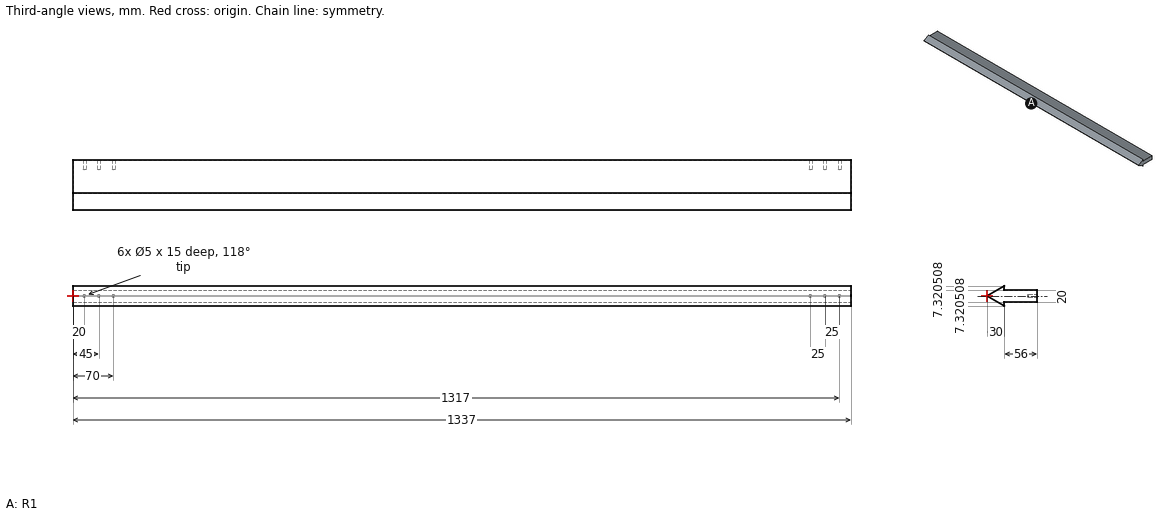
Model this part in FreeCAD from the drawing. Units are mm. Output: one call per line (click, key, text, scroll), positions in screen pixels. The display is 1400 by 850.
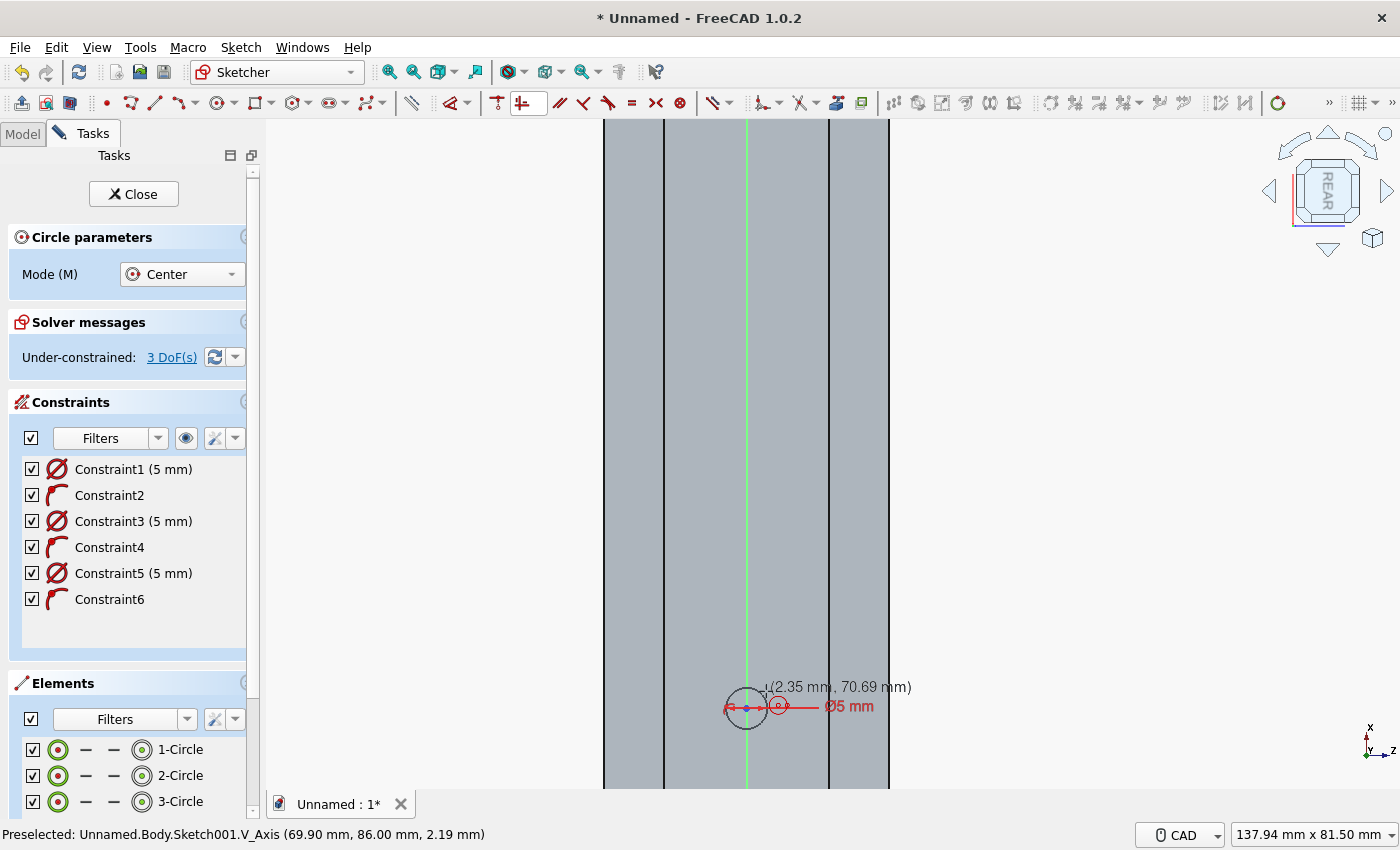
scroll(765, 695, down, 15)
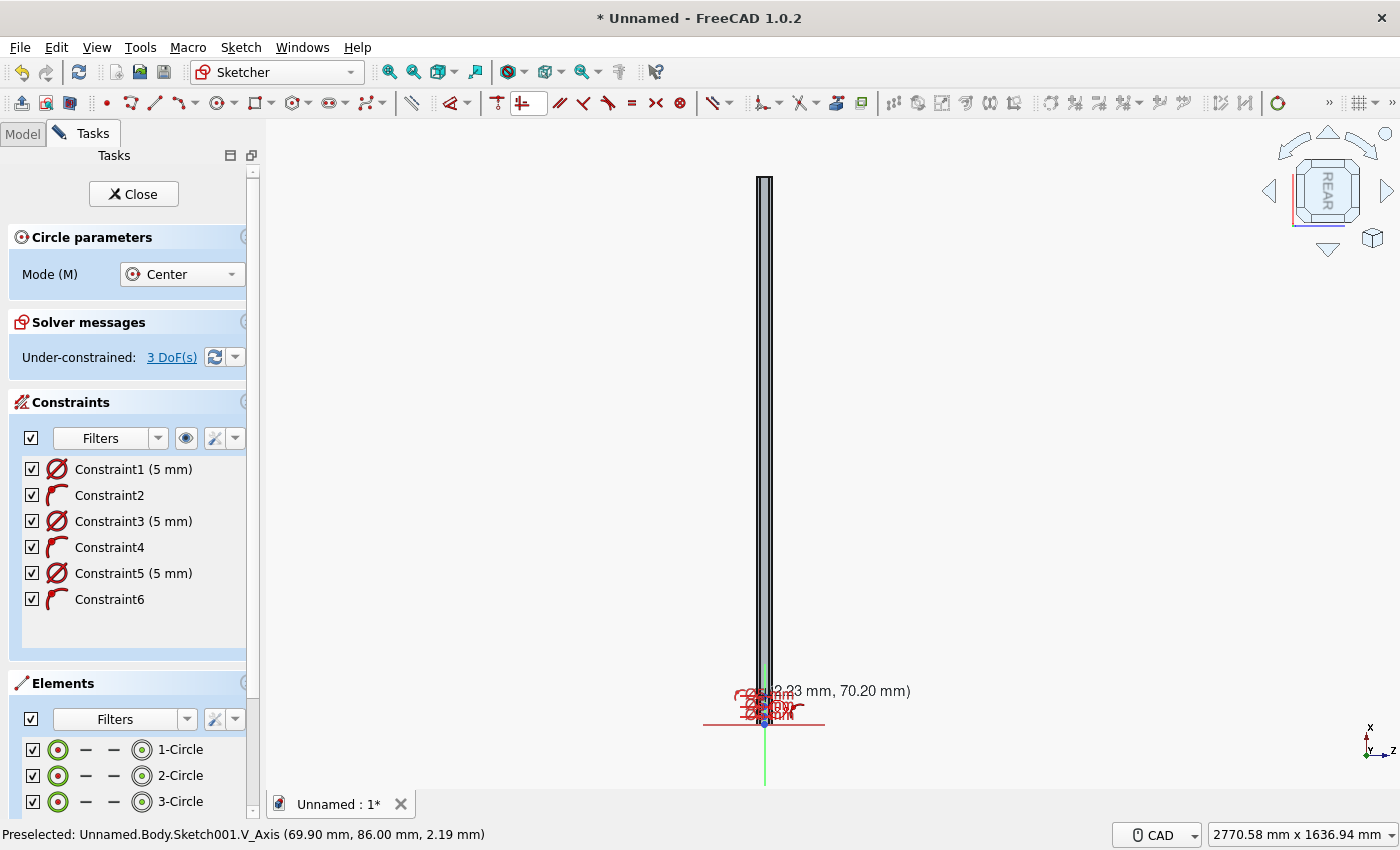
scroll(765, 186, up, 16)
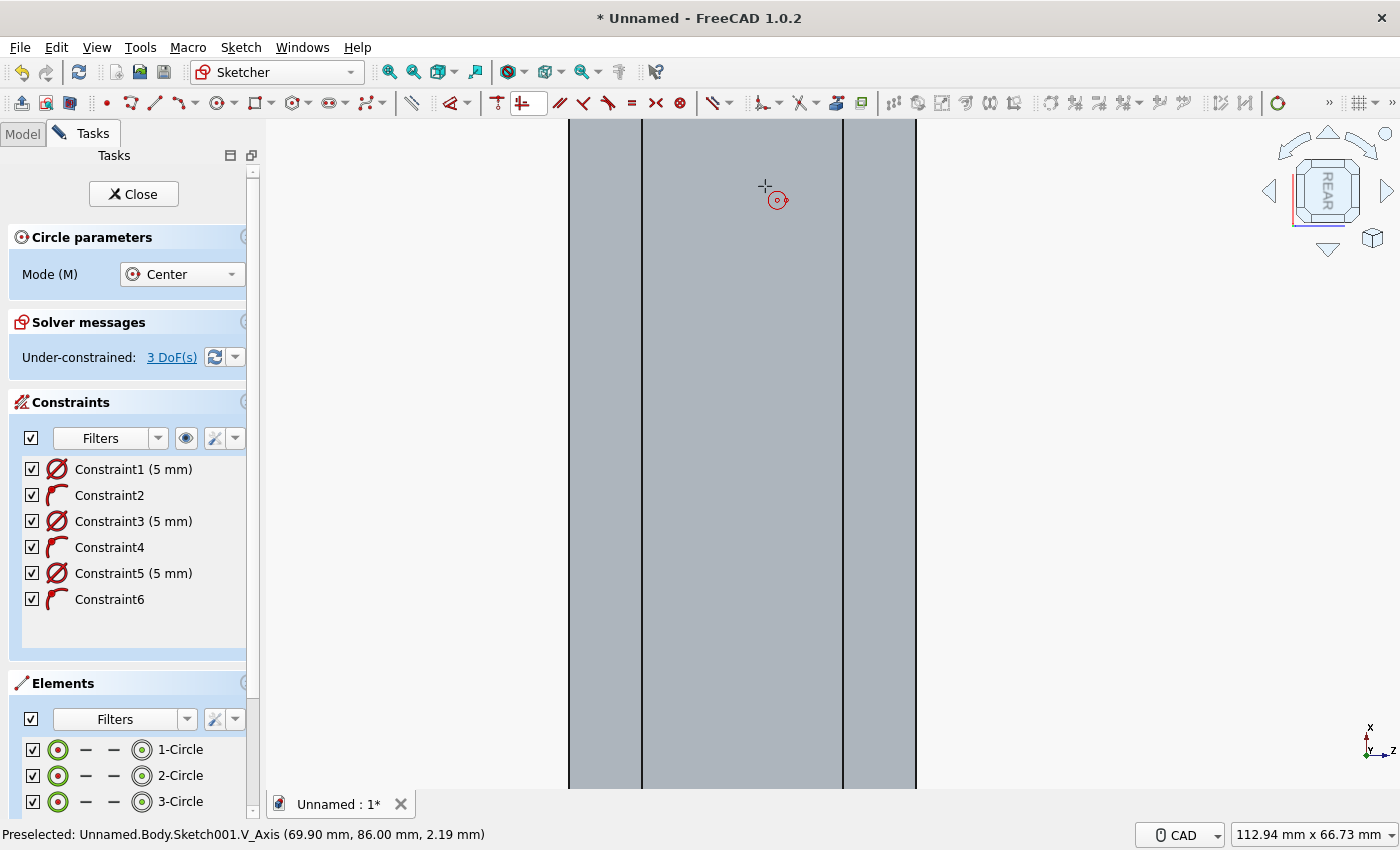
scroll(765, 186, down, 16)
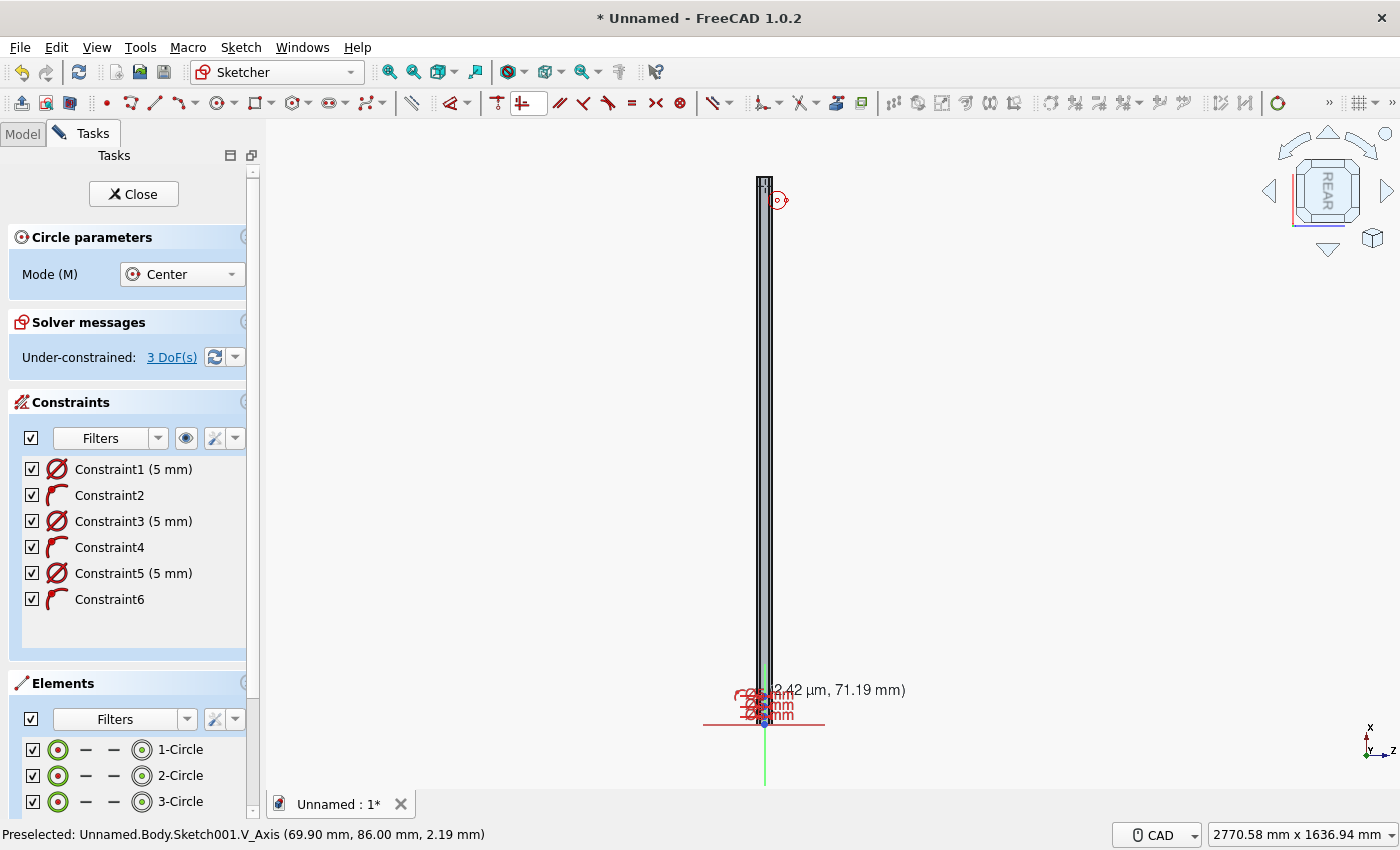
click(765, 186)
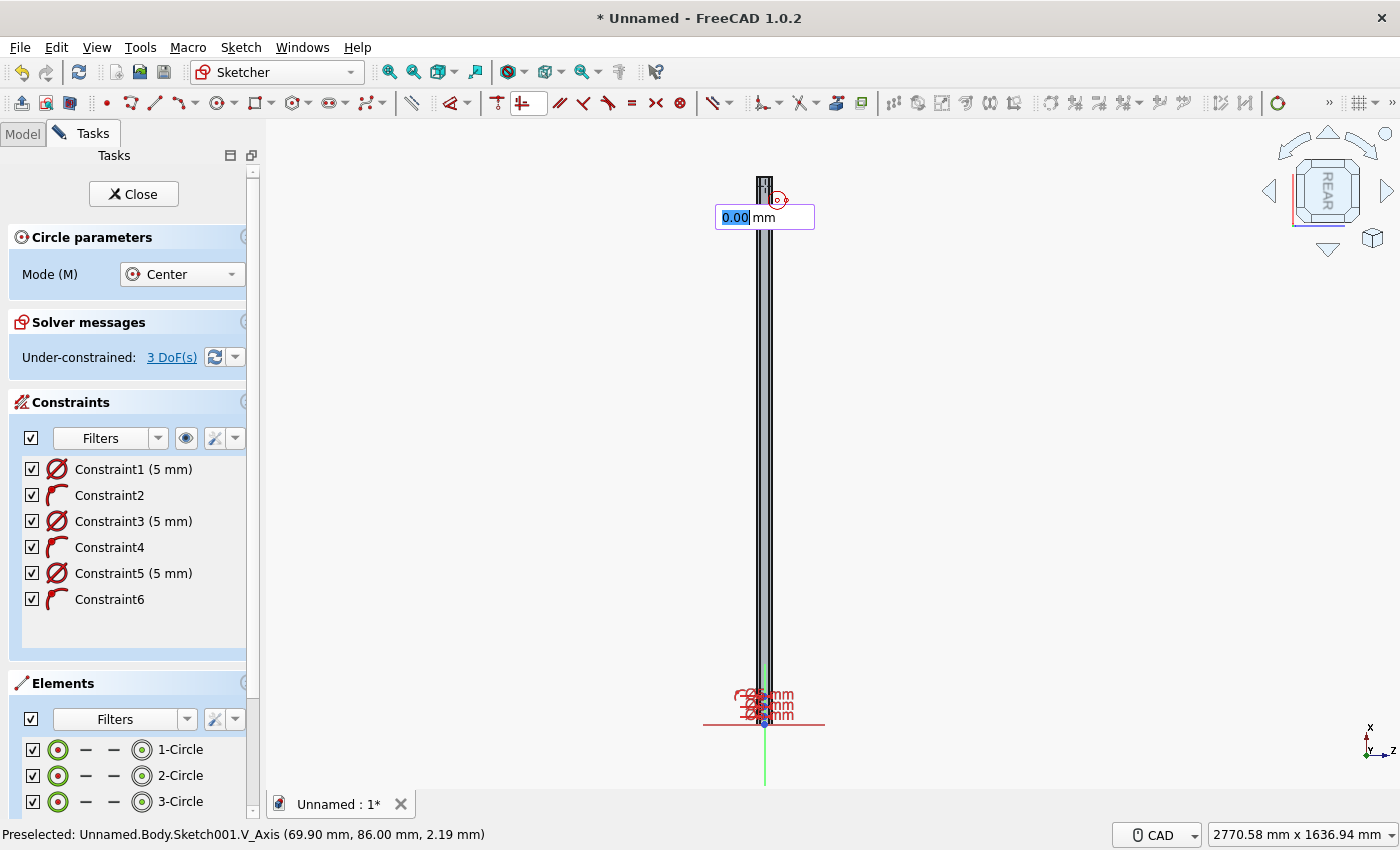
scroll(765, 185, up, 15)
move(766, 187)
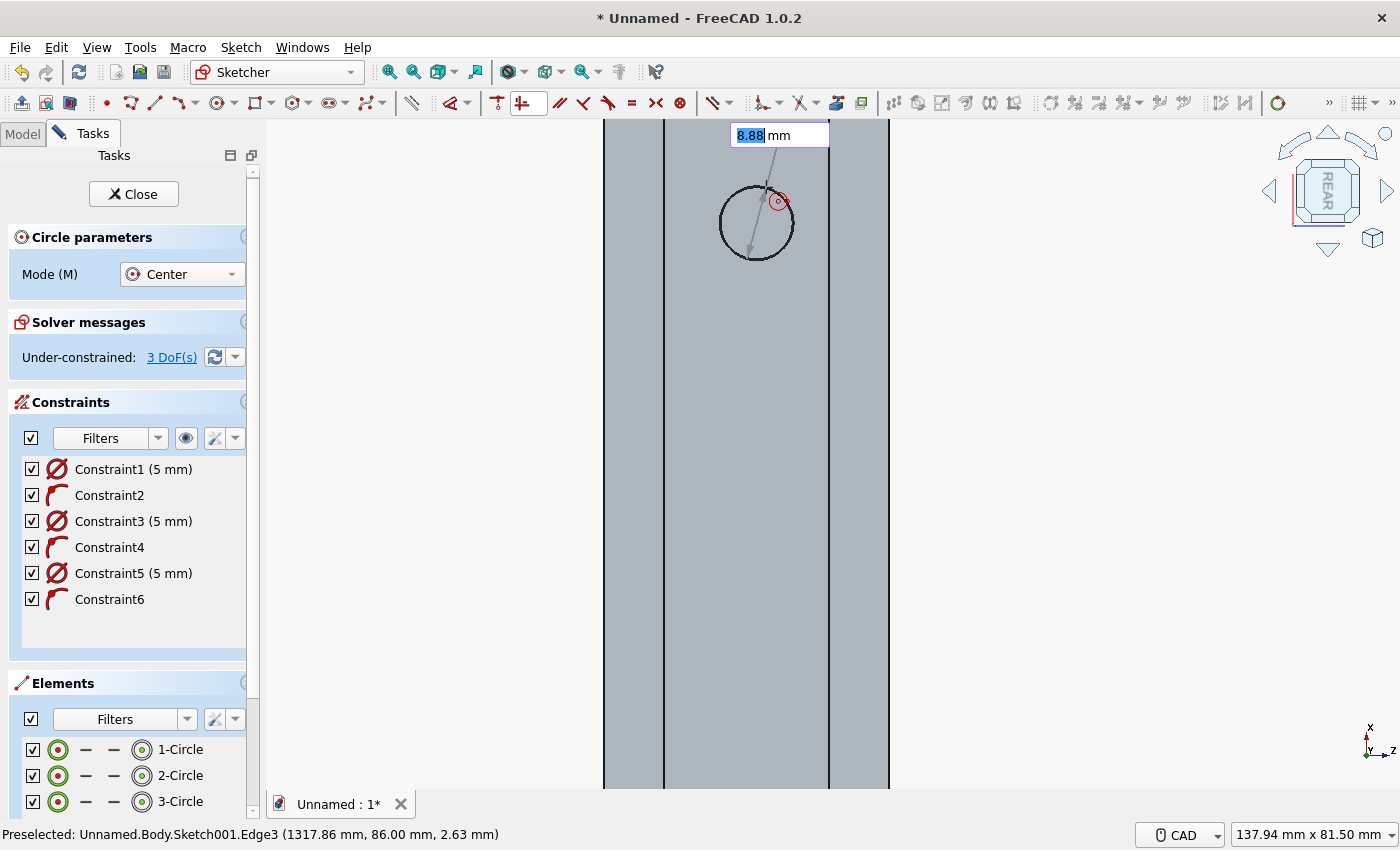
text(5)
key(Return)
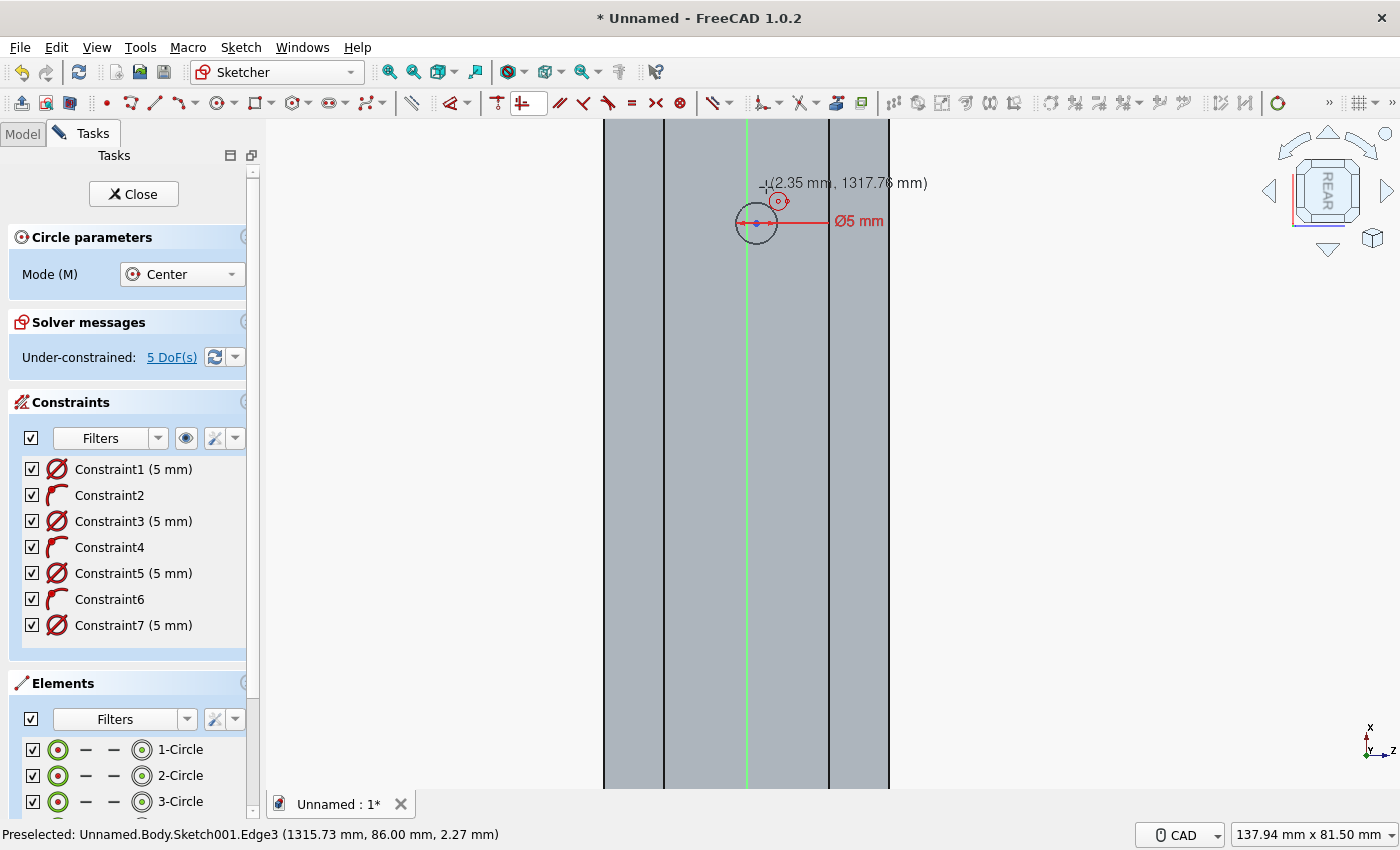
scroll(765, 185, down, 15)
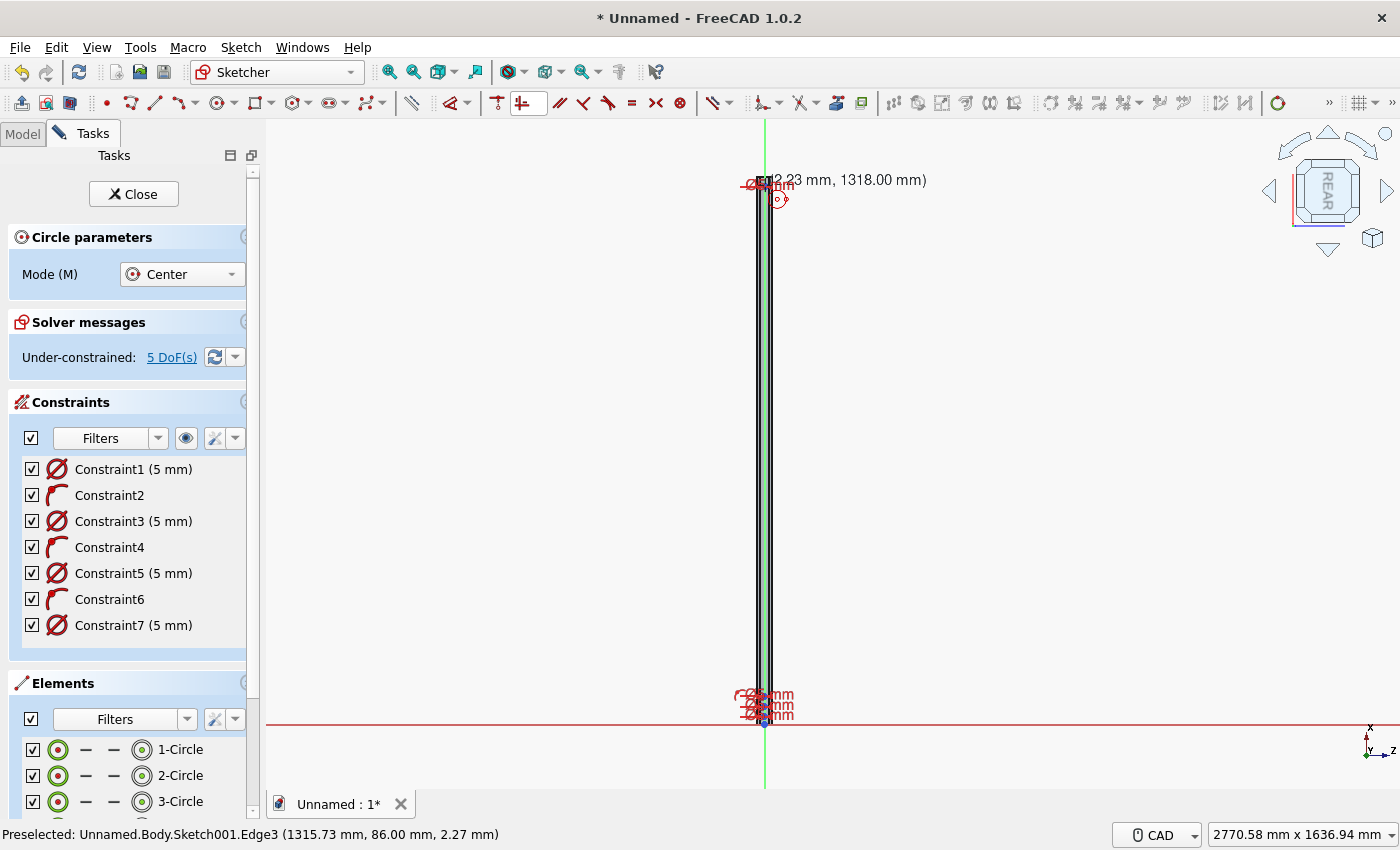
scroll(765, 196, up, 3)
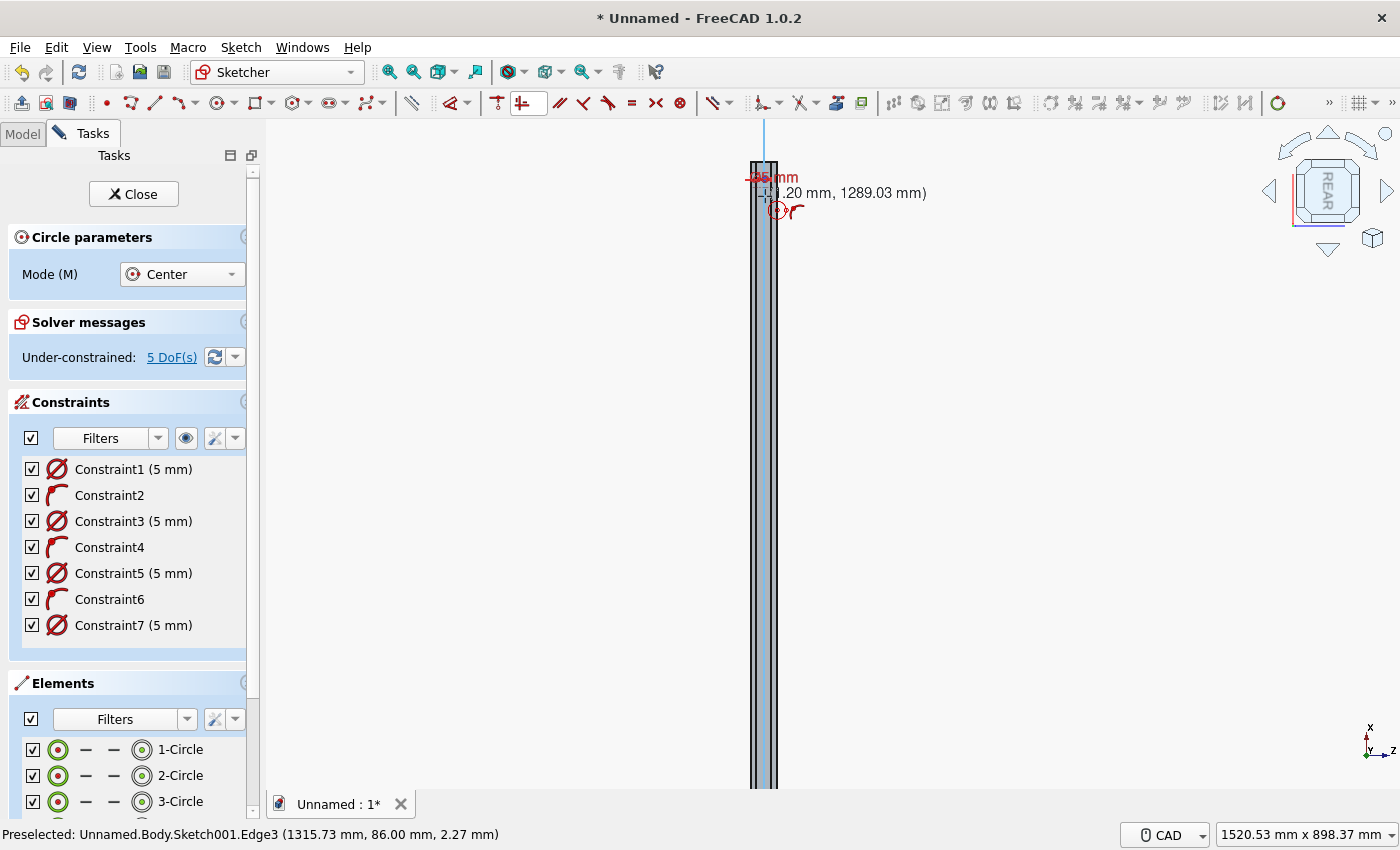
click(764, 196)